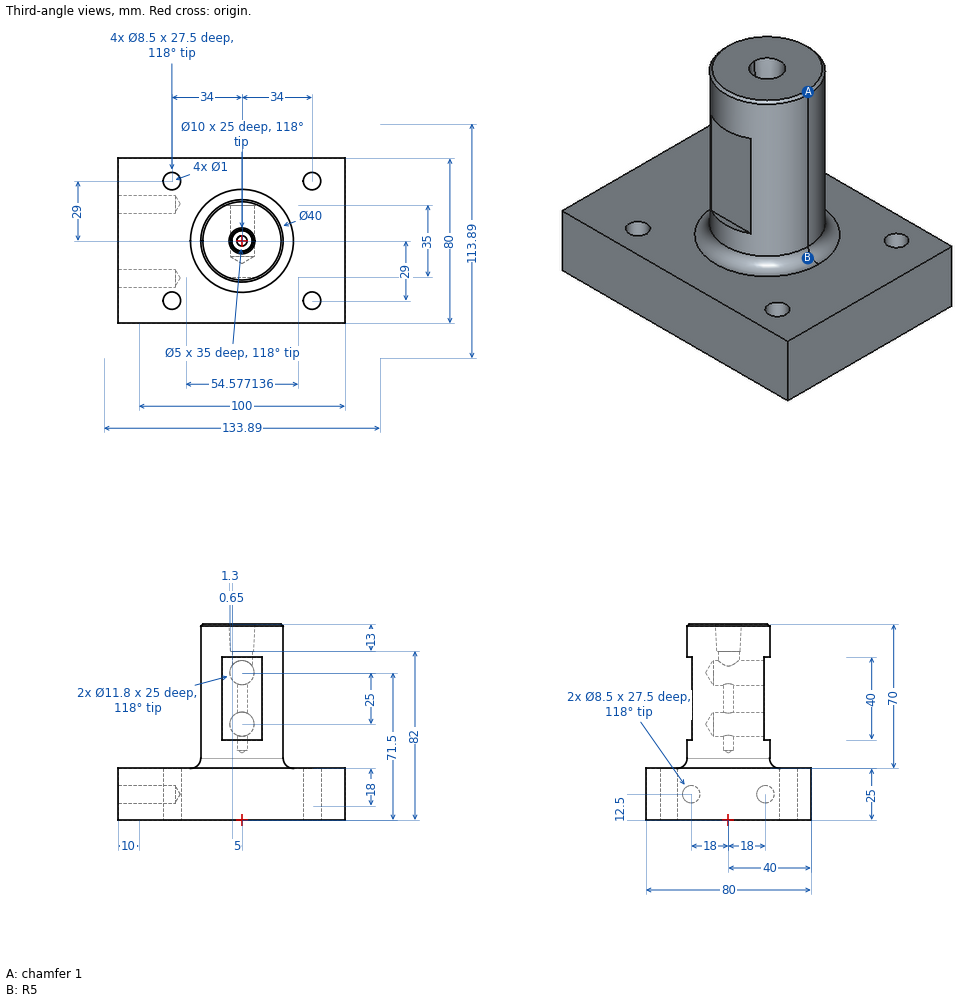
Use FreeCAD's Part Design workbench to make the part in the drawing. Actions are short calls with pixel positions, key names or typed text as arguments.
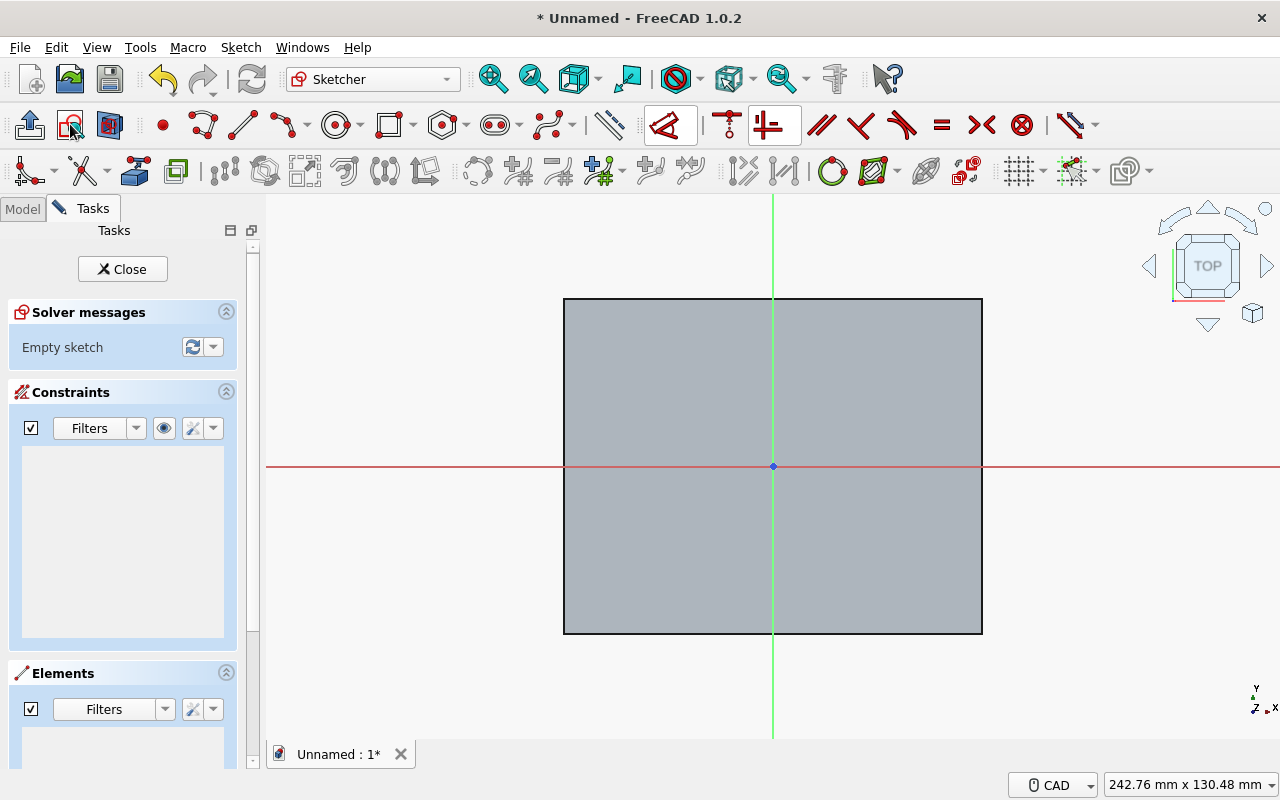
scroll(912, 467, up, 2)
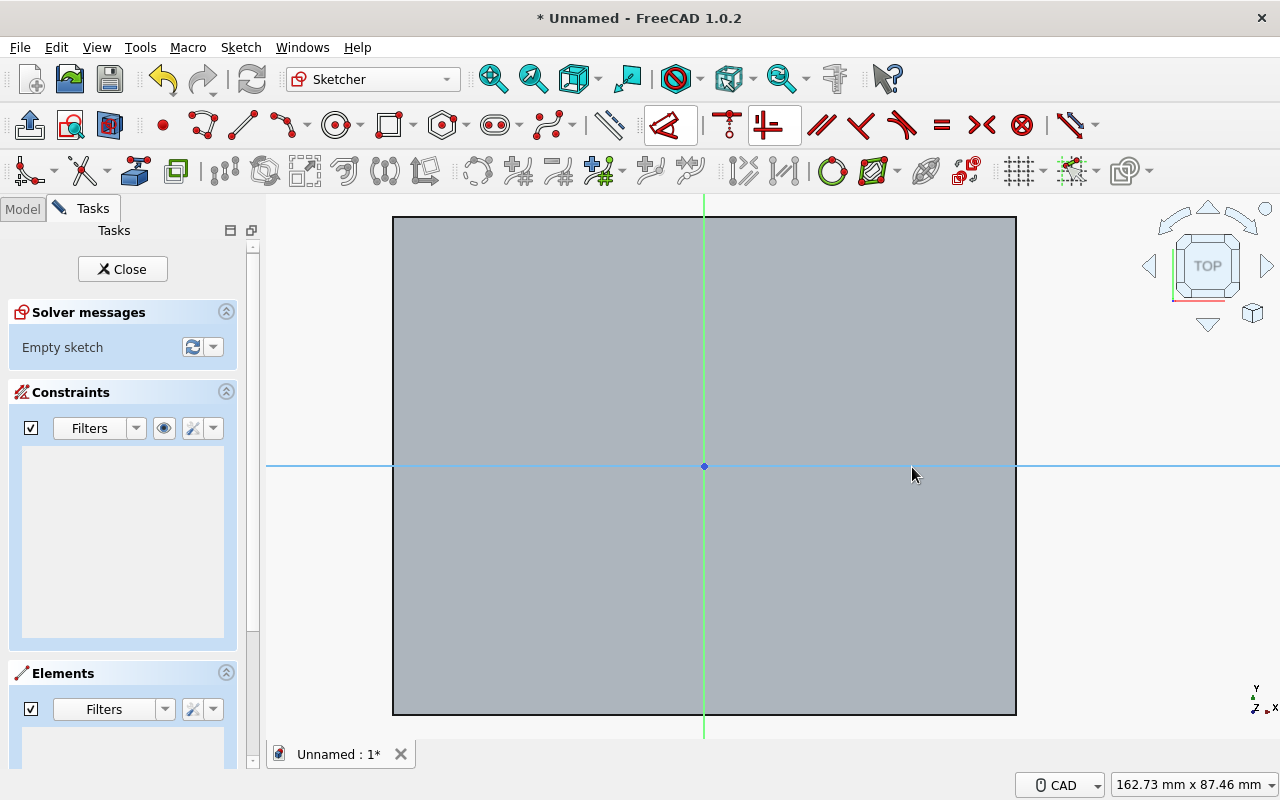
key(g)
key(c)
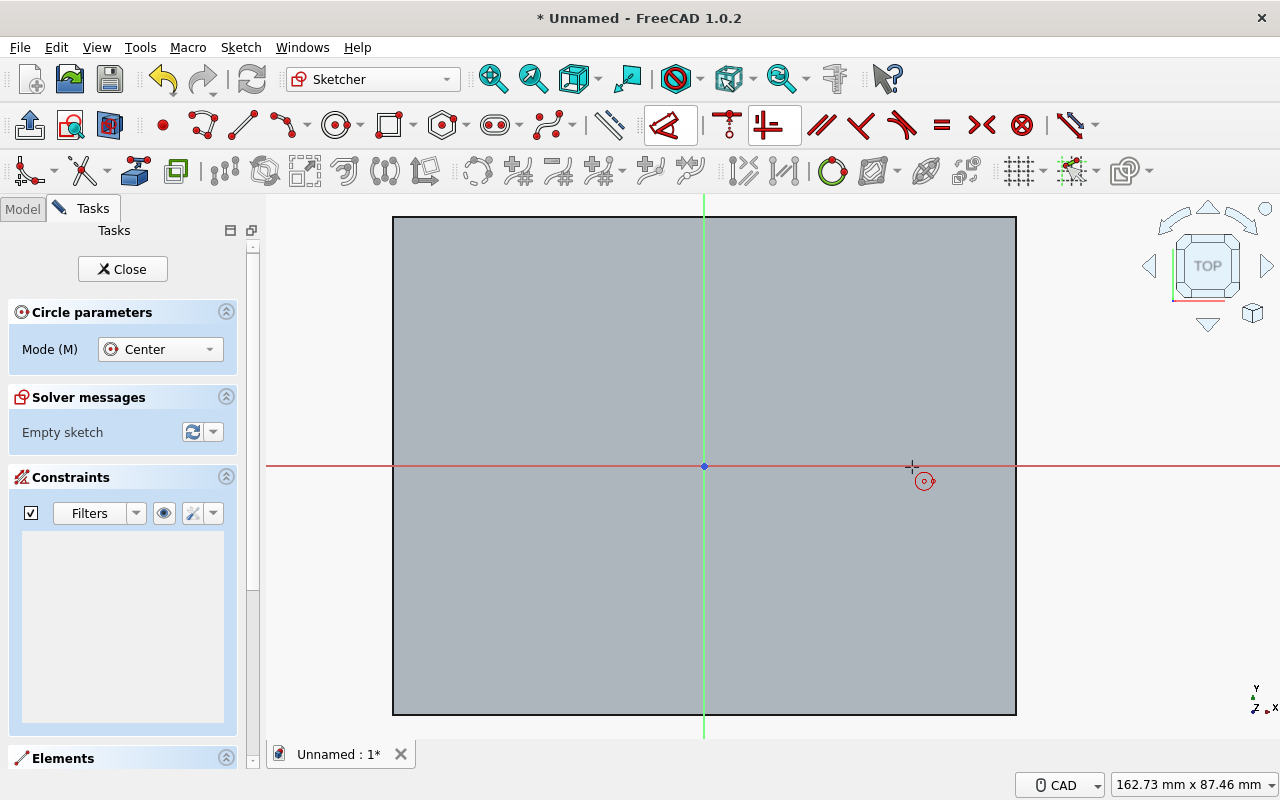
scroll(492, 285, up, 10)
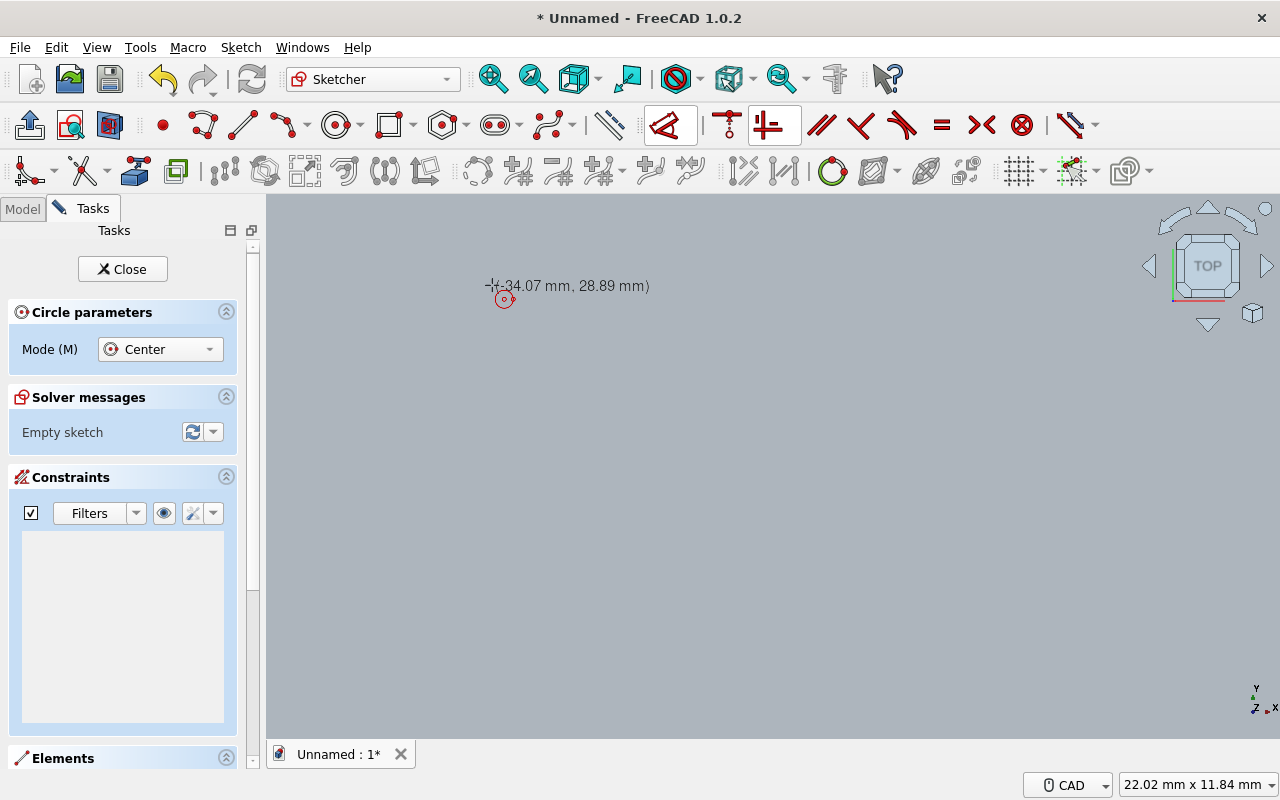
scroll(492, 286, down, 10)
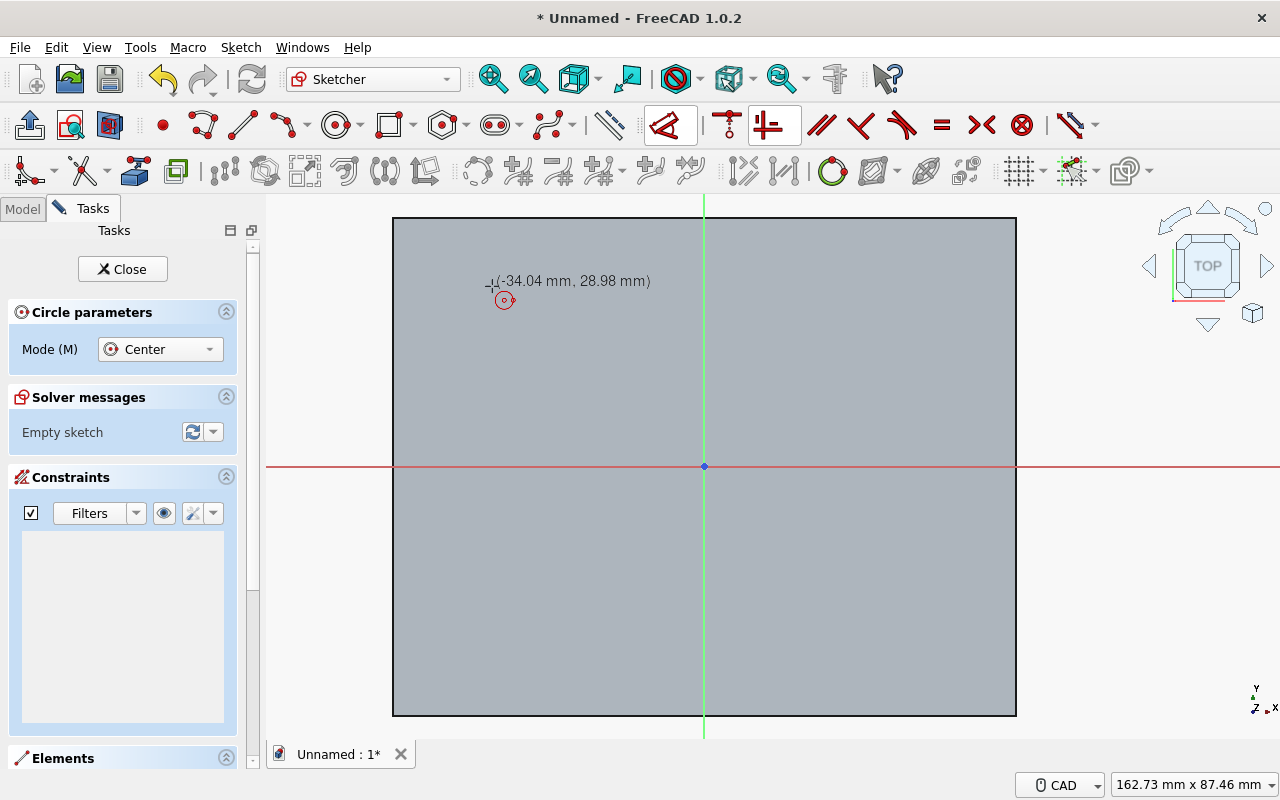
click(492, 286)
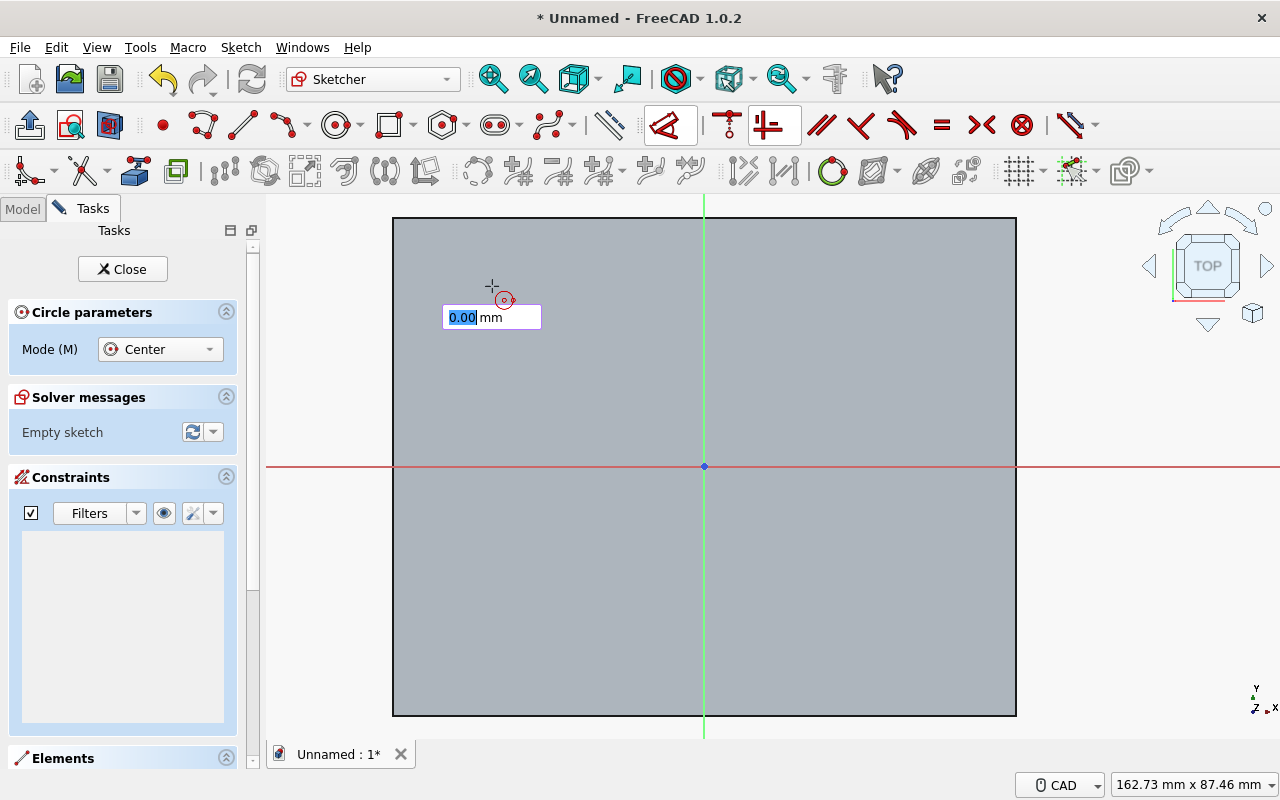
scroll(495, 284, up, 9)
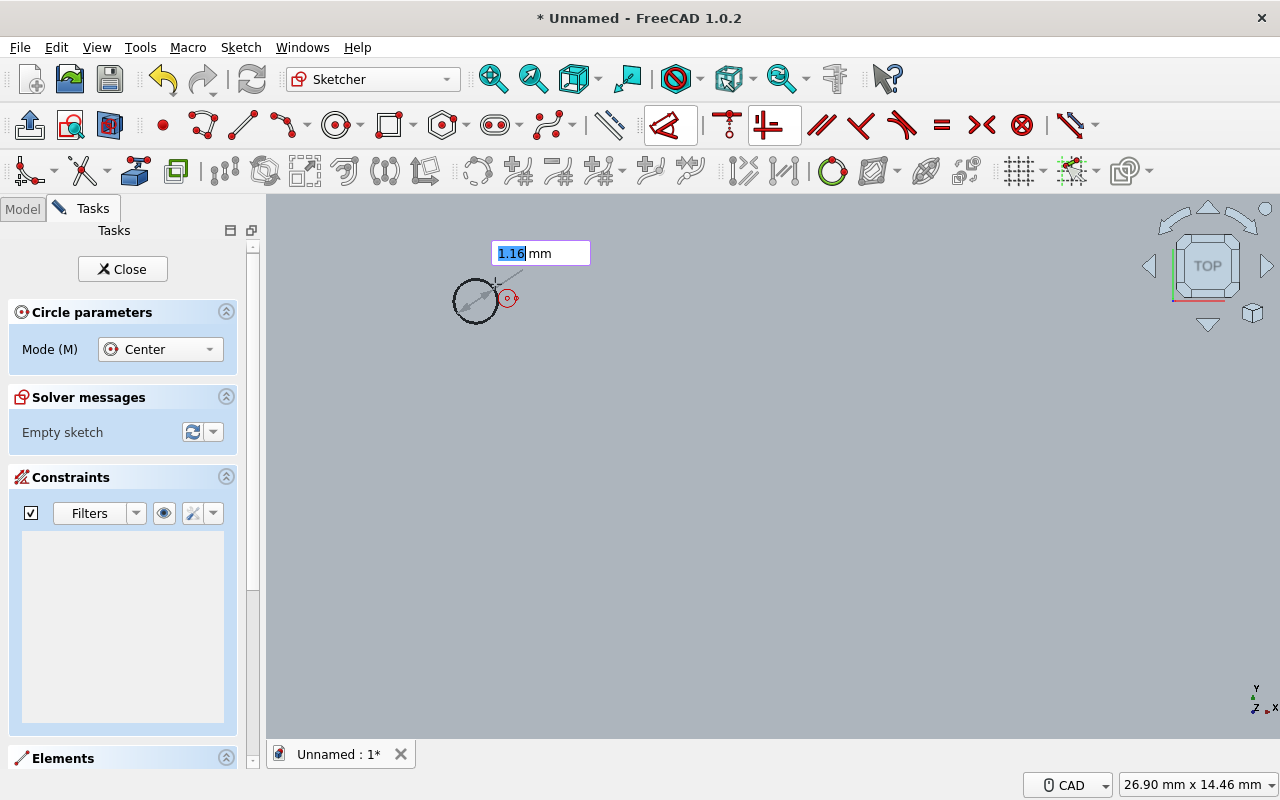
click(492, 283)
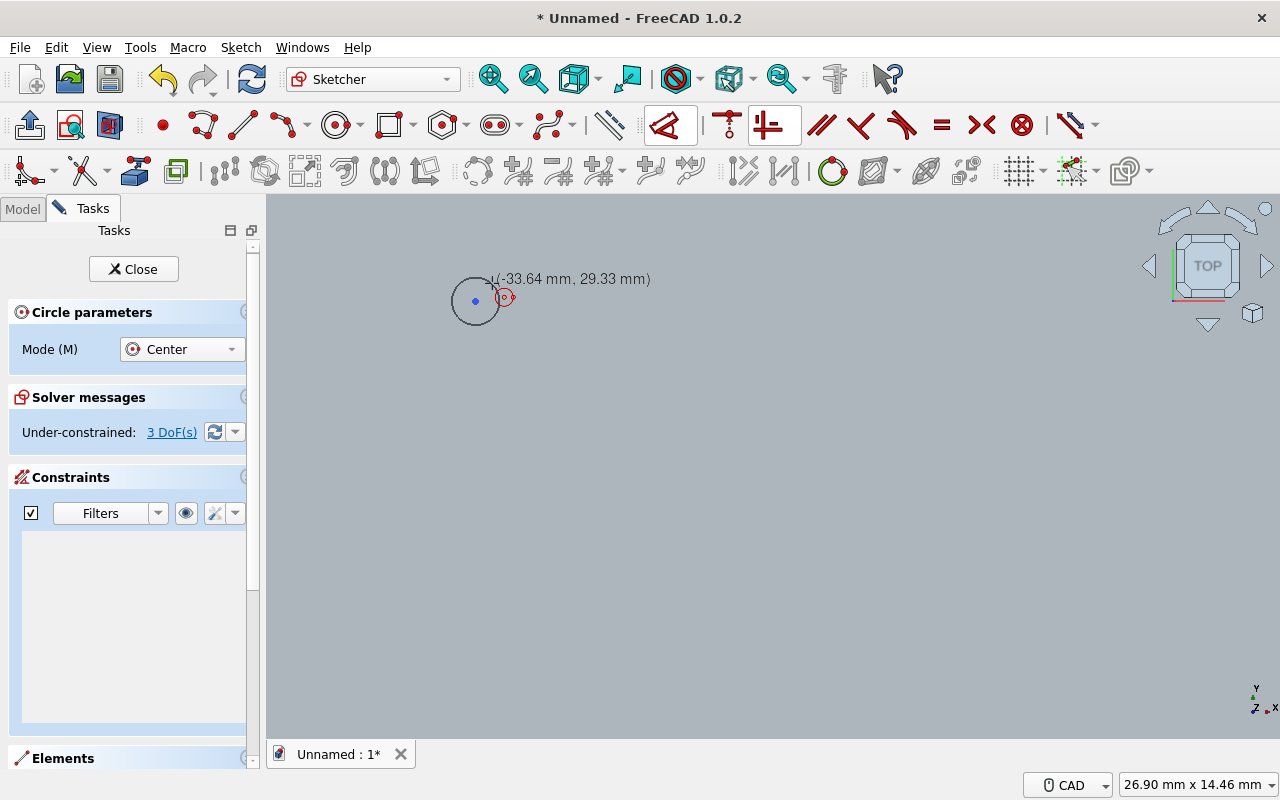
scroll(495, 284, down, 9)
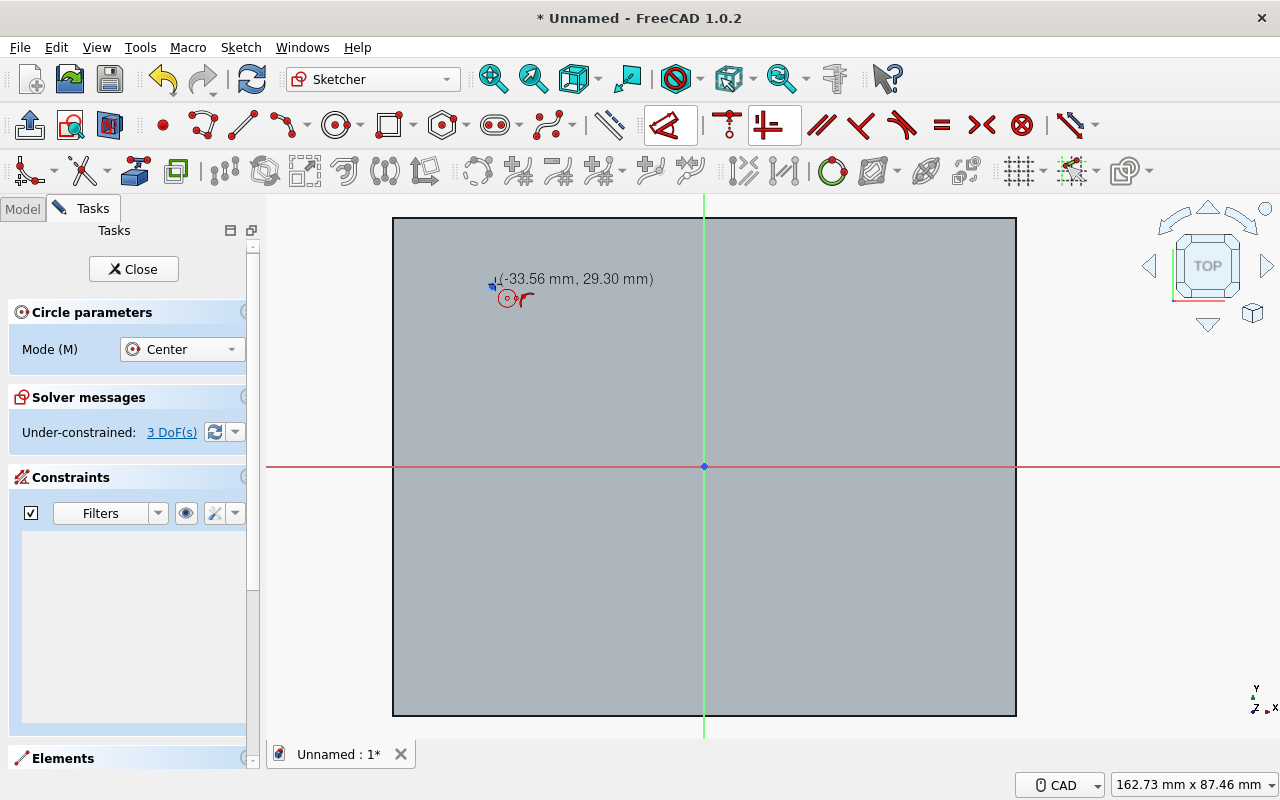
scroll(916, 286, up, 10)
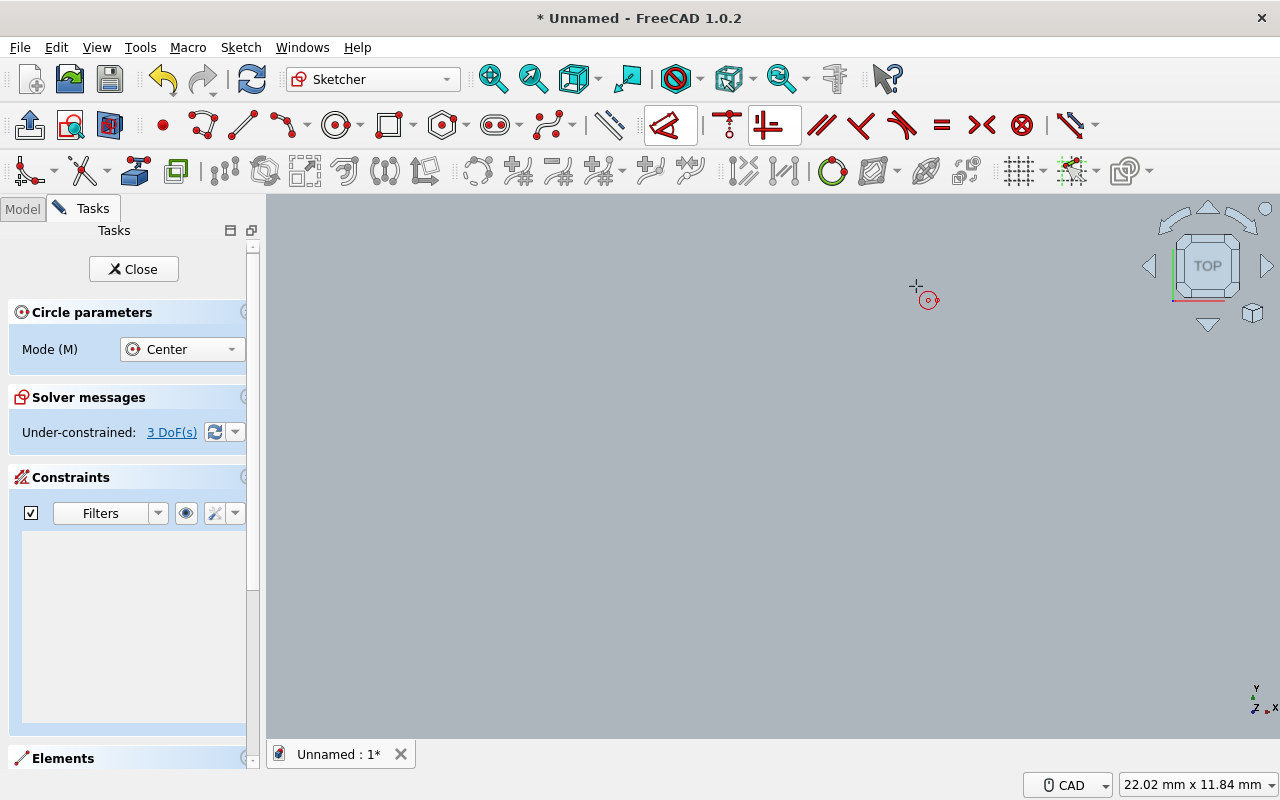
scroll(917, 286, down, 10)